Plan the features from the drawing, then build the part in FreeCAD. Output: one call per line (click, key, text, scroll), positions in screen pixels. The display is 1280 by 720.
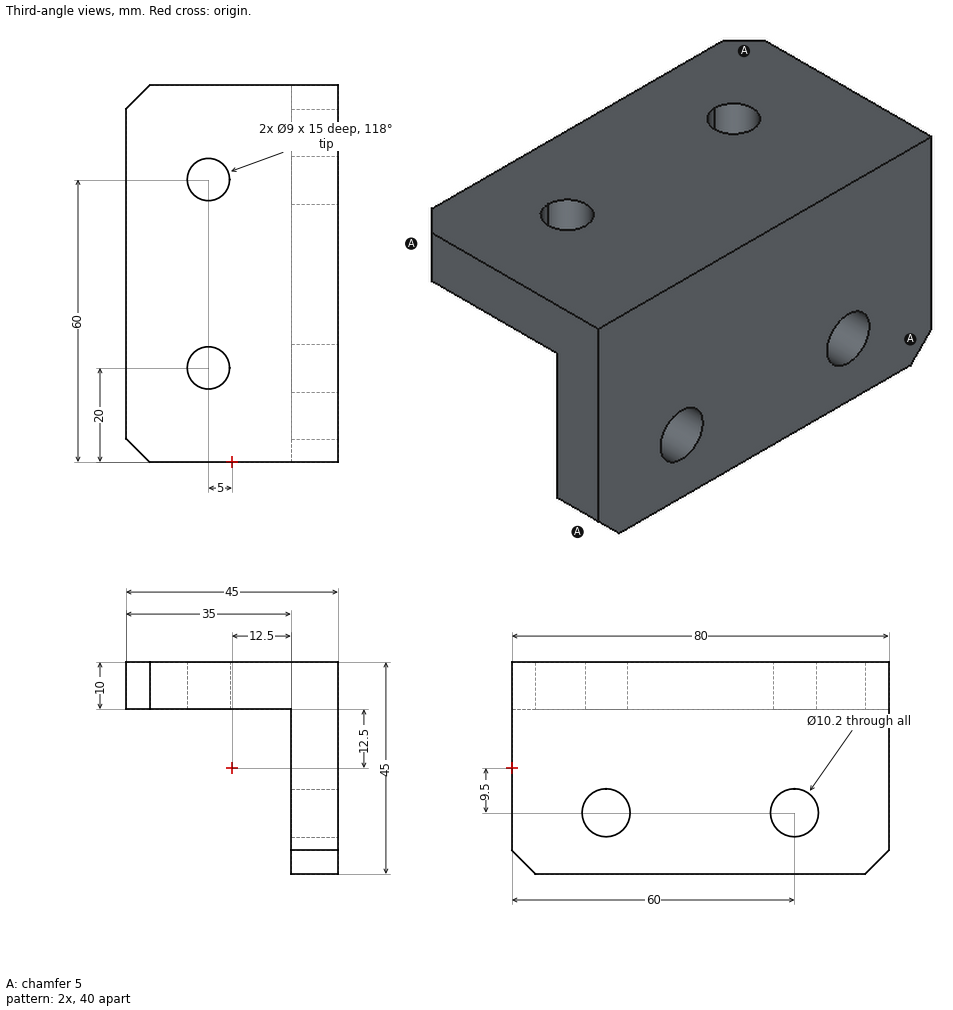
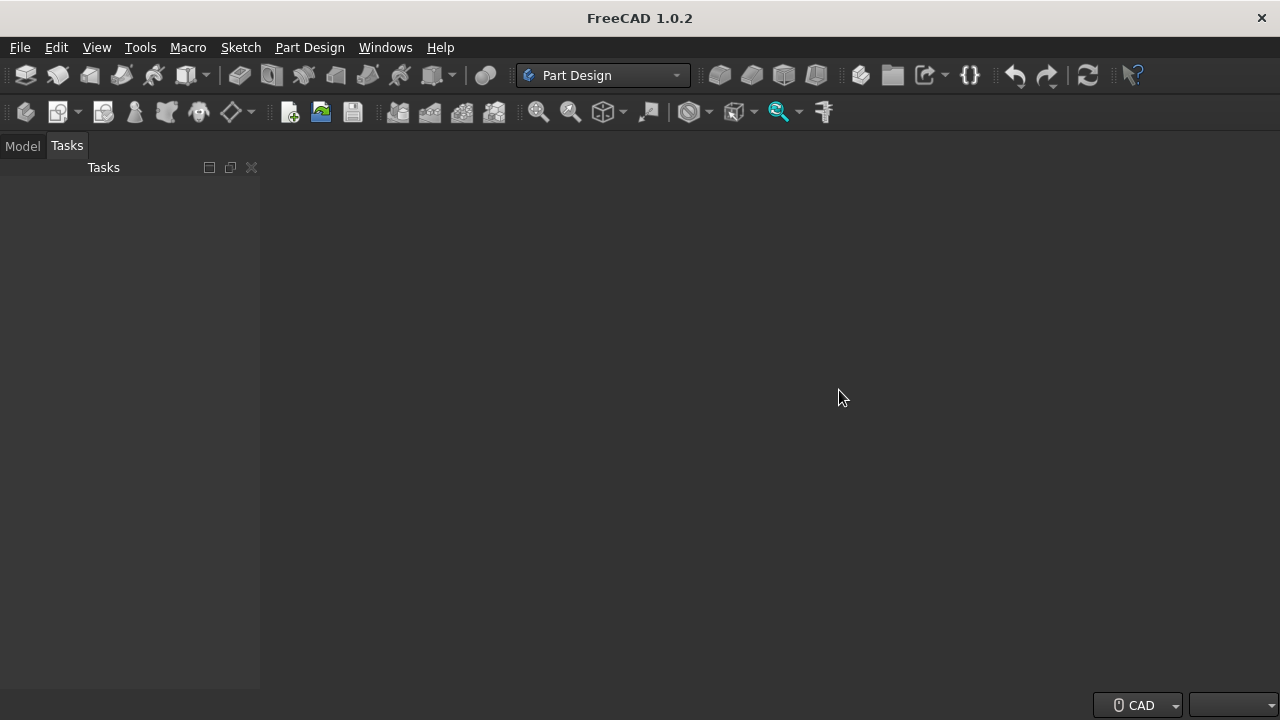
key(ctrl+n)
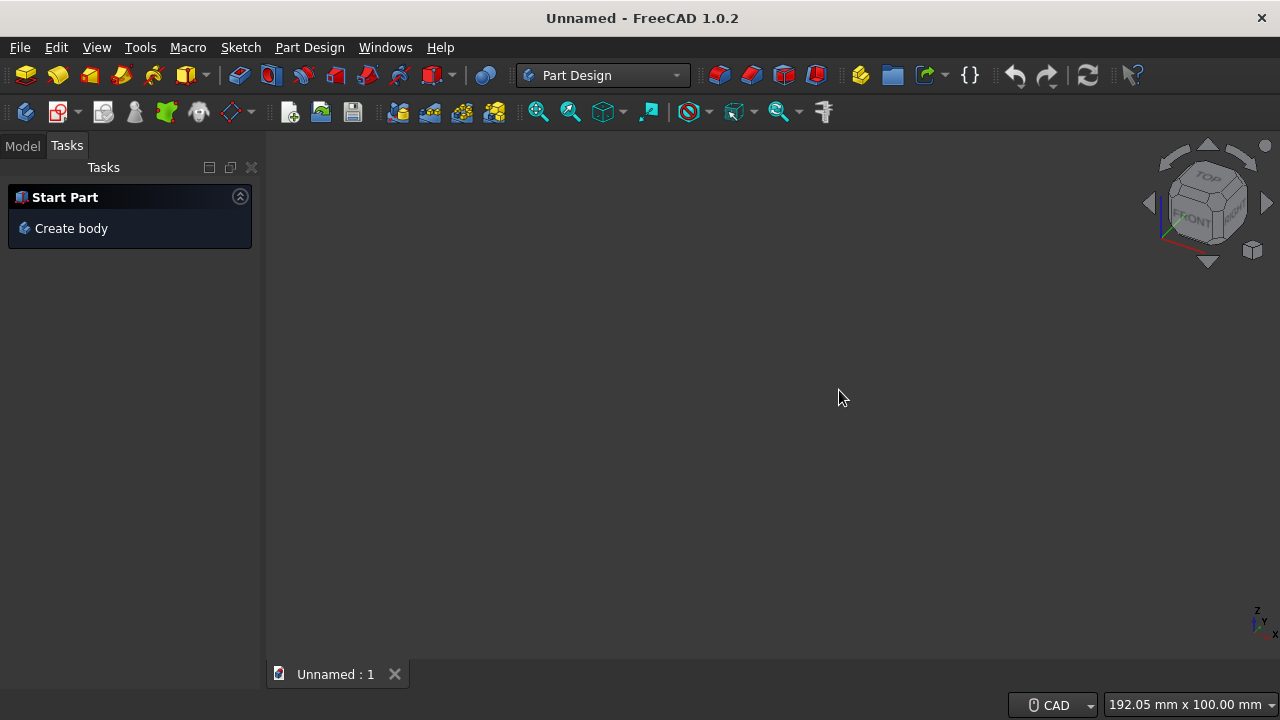
click(58, 112)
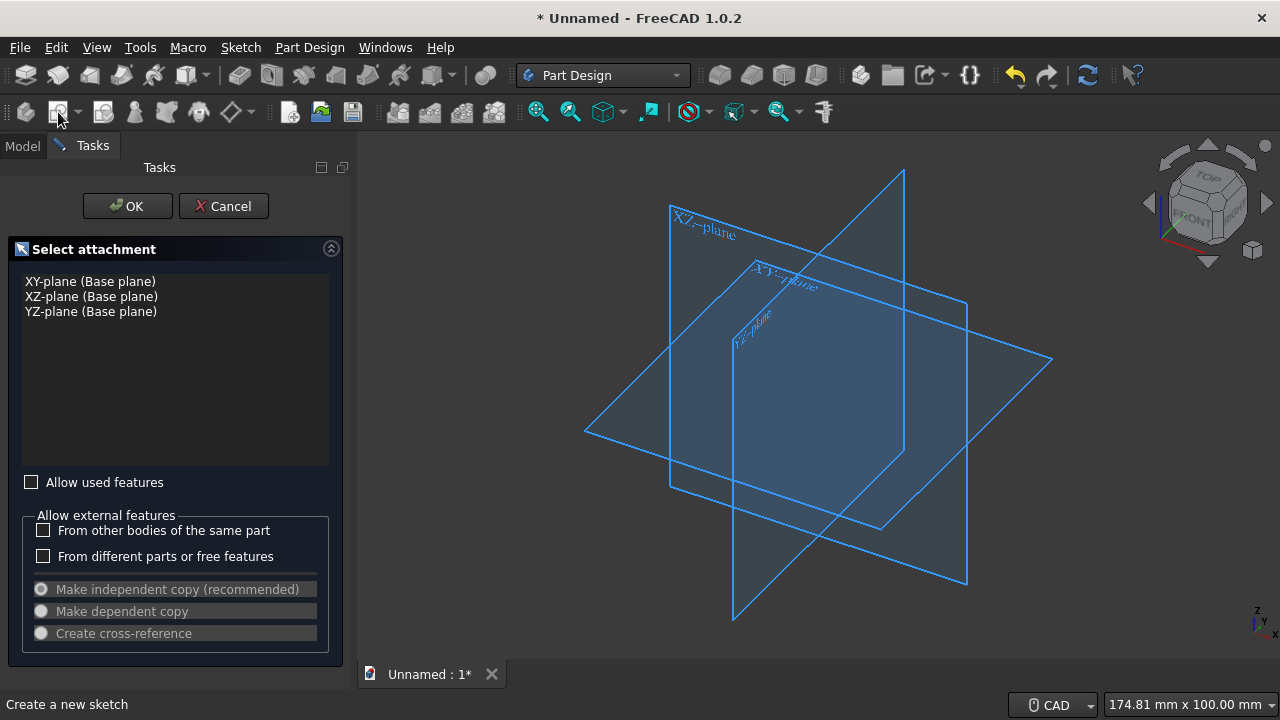
click(82, 296)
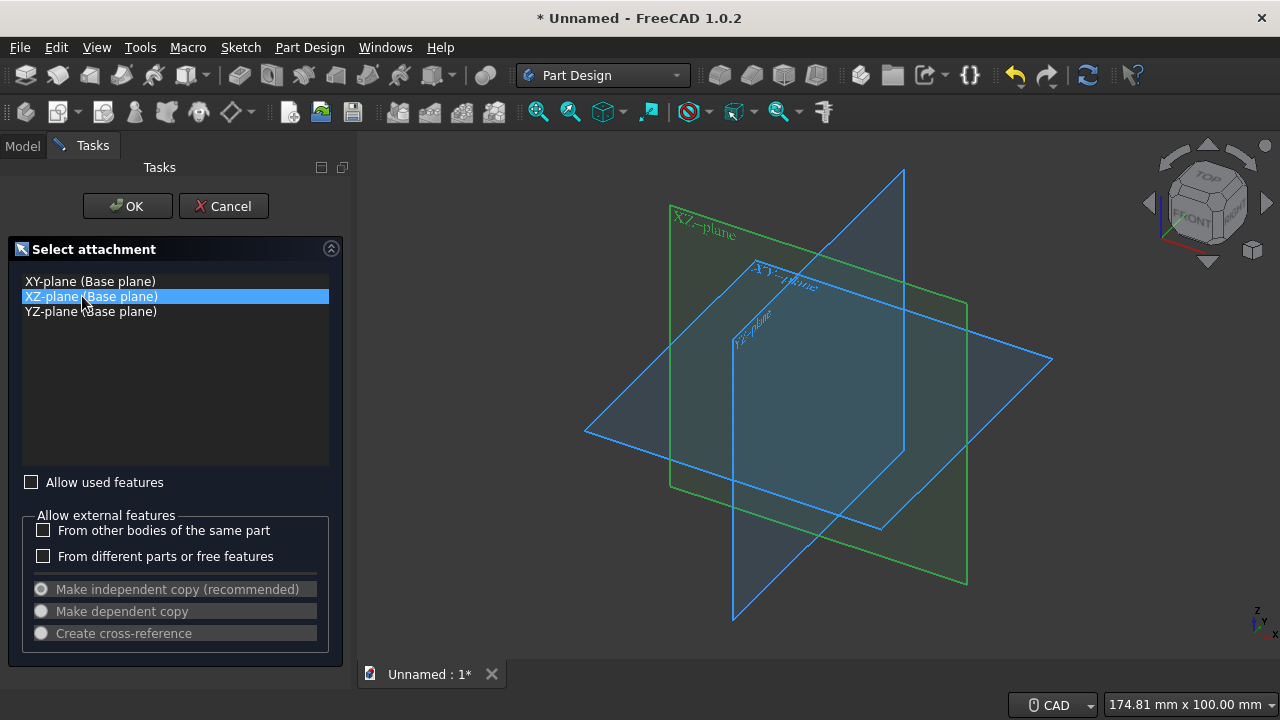
click(128, 206)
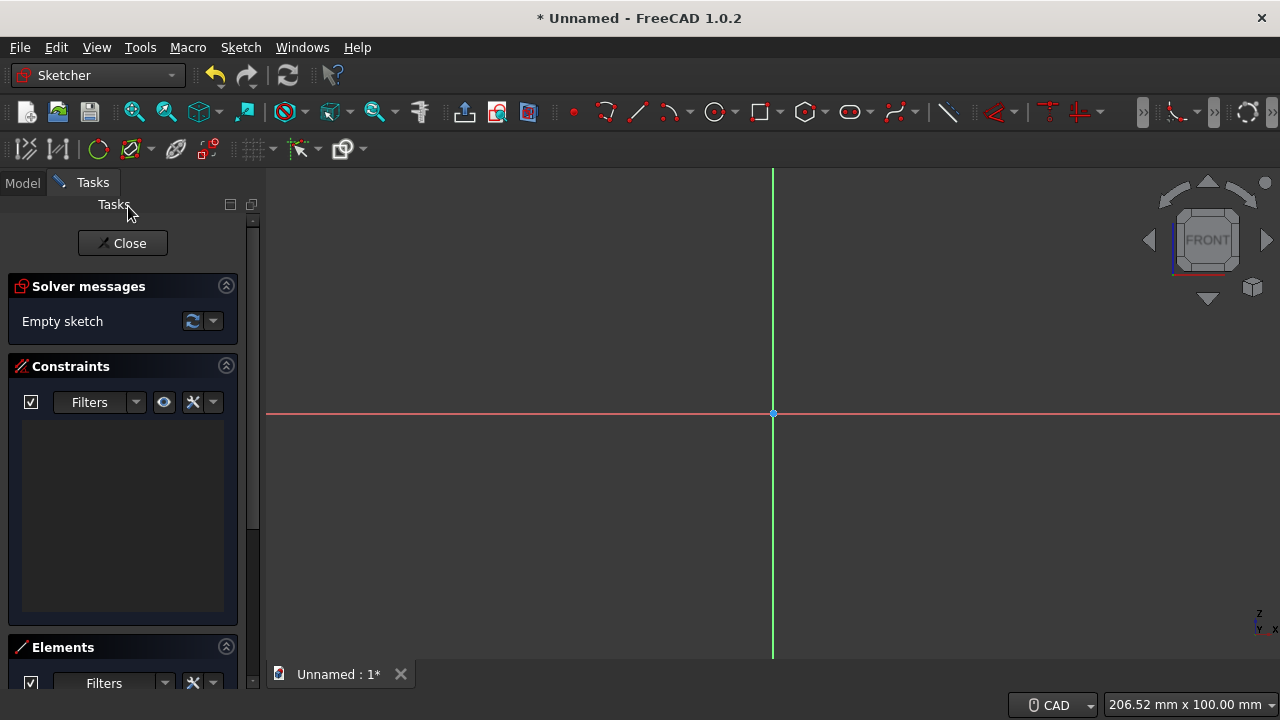
scroll(912, 413, up, 2)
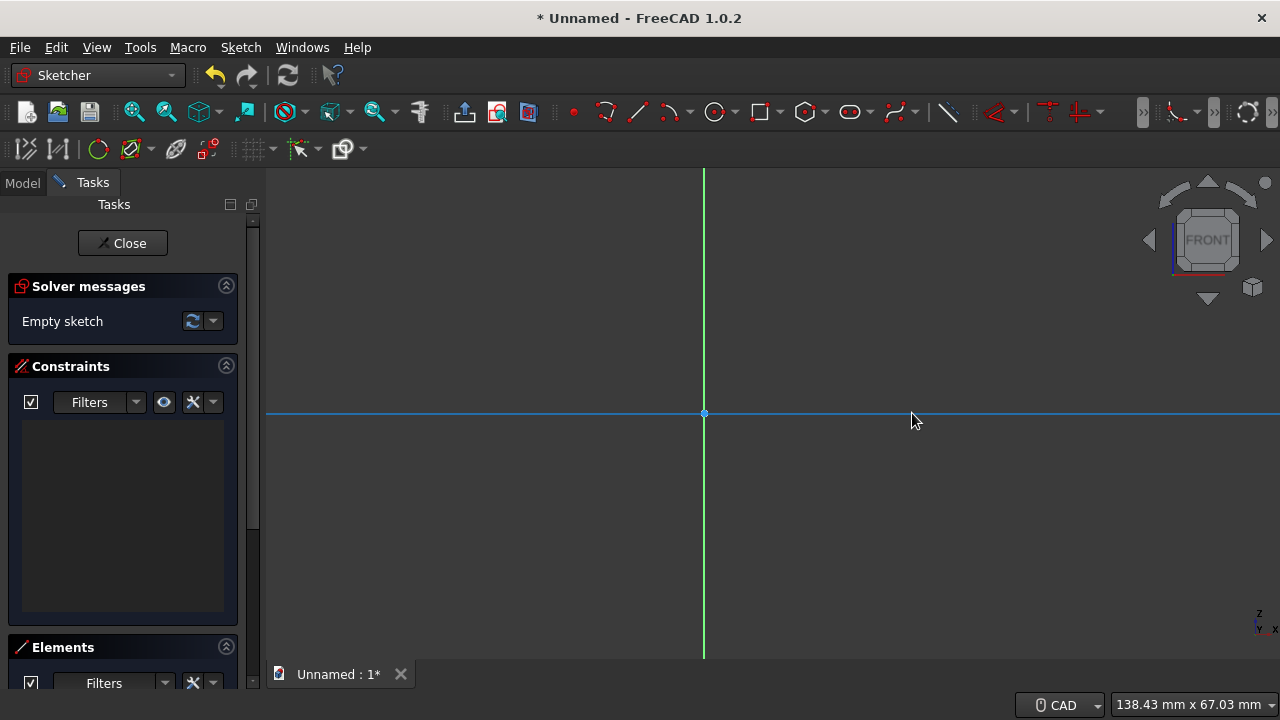
key(g)
key(m)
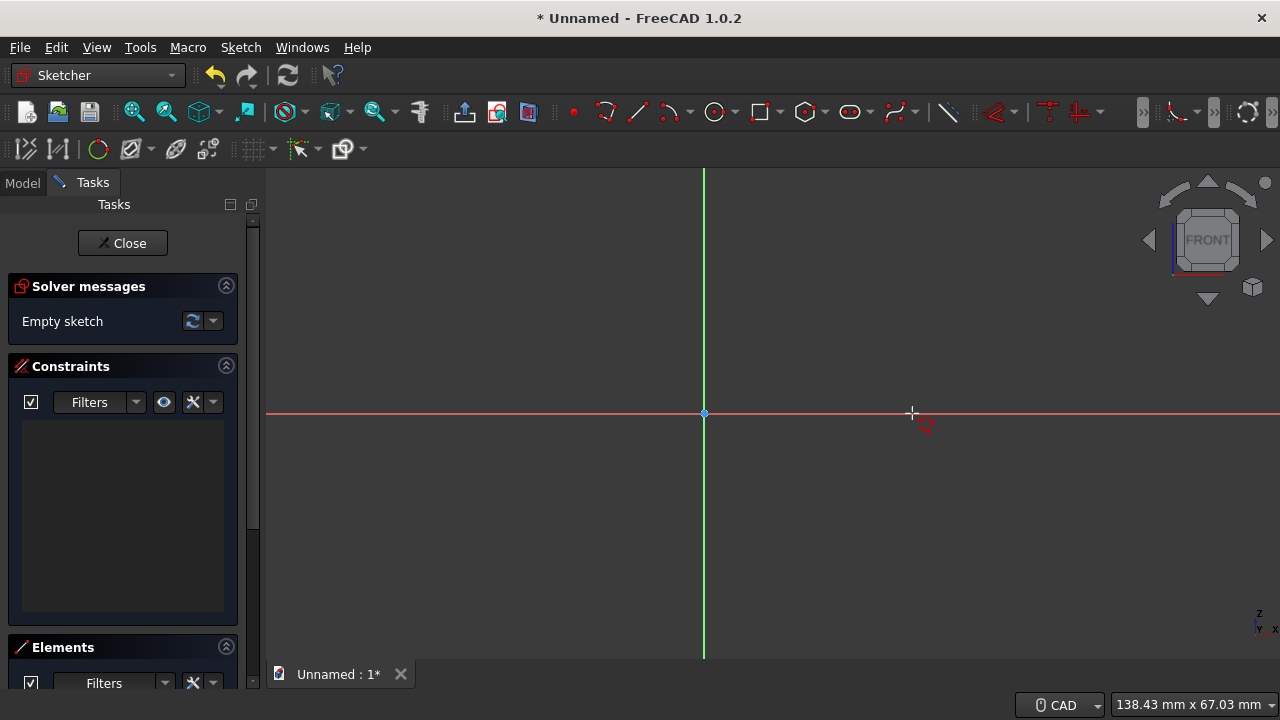
click(796, 322)
click(540, 322)
click(540, 249)
click(869, 249)
click(869, 578)
click(796, 578)
click(796, 323)
key(Escape)
key(Escape)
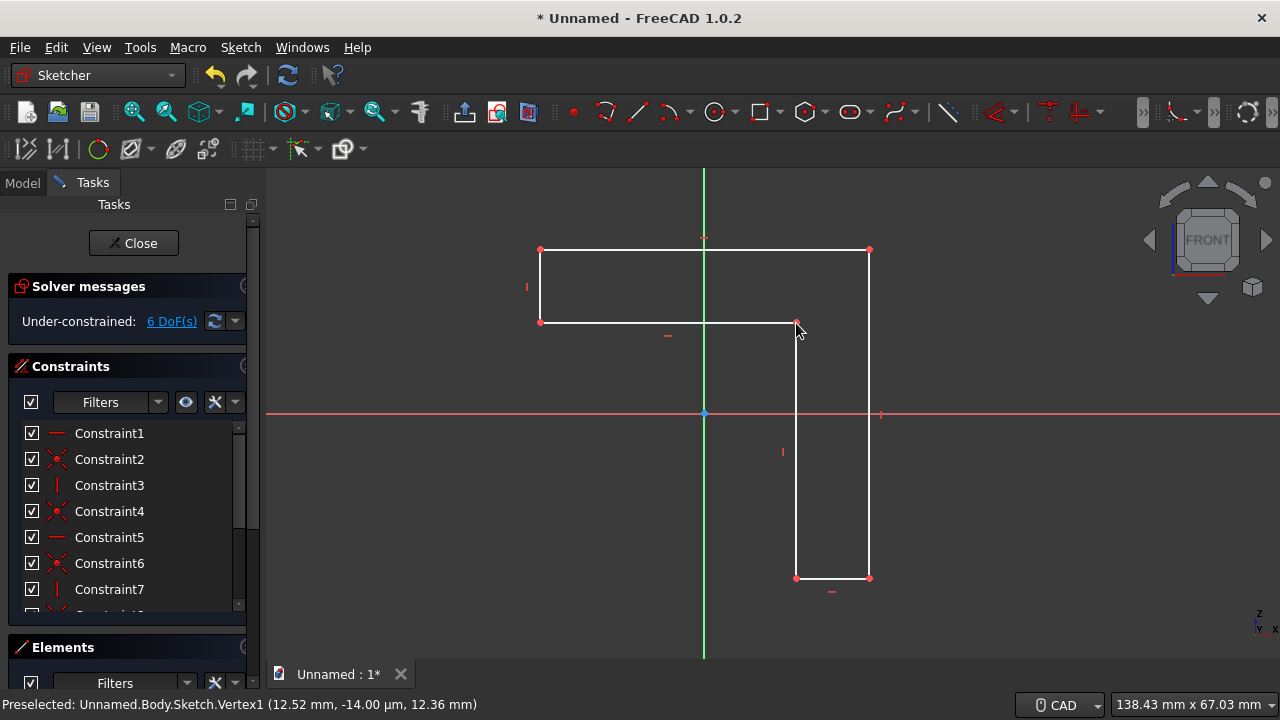
click(994, 112)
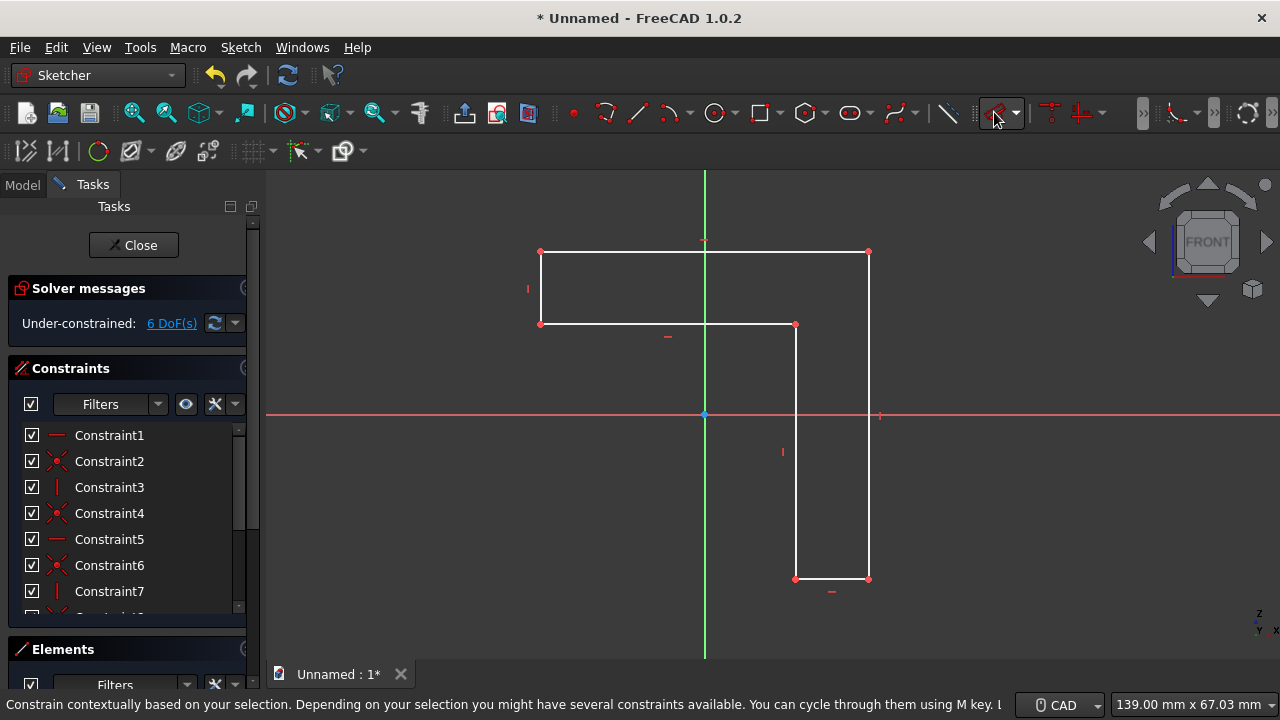
click(719, 324)
click(668, 290)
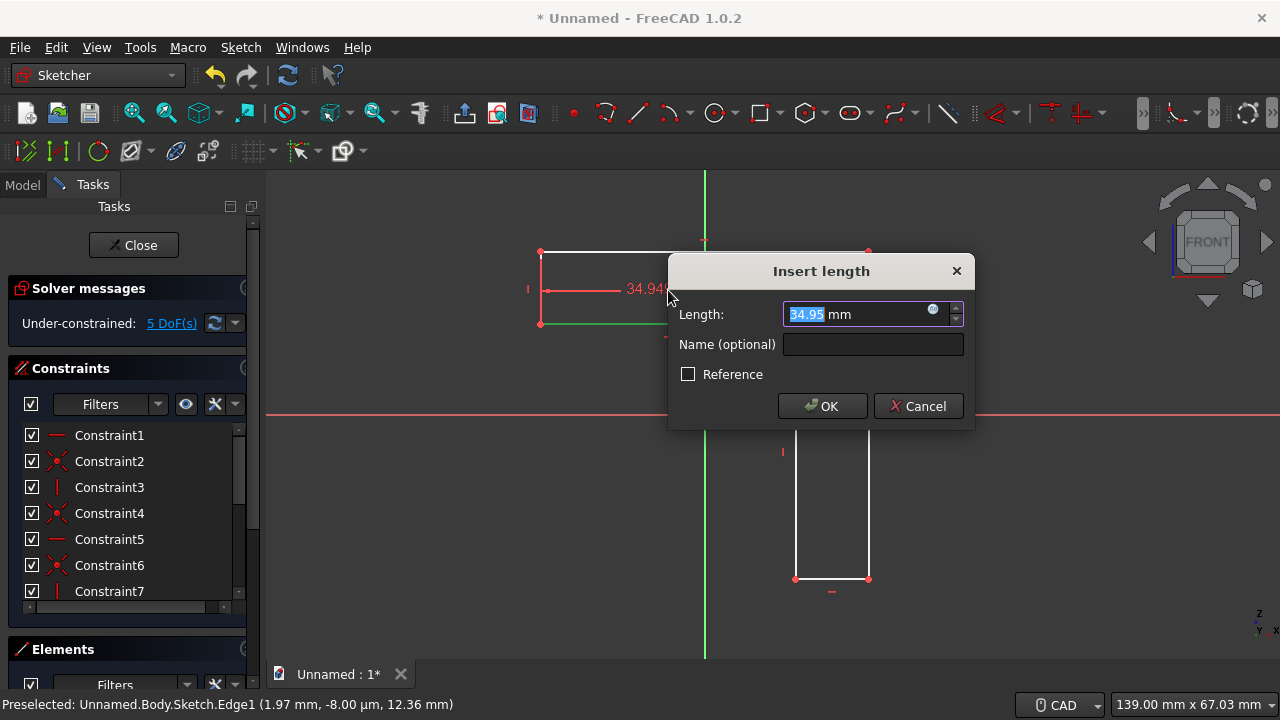
text(35)
key(Return)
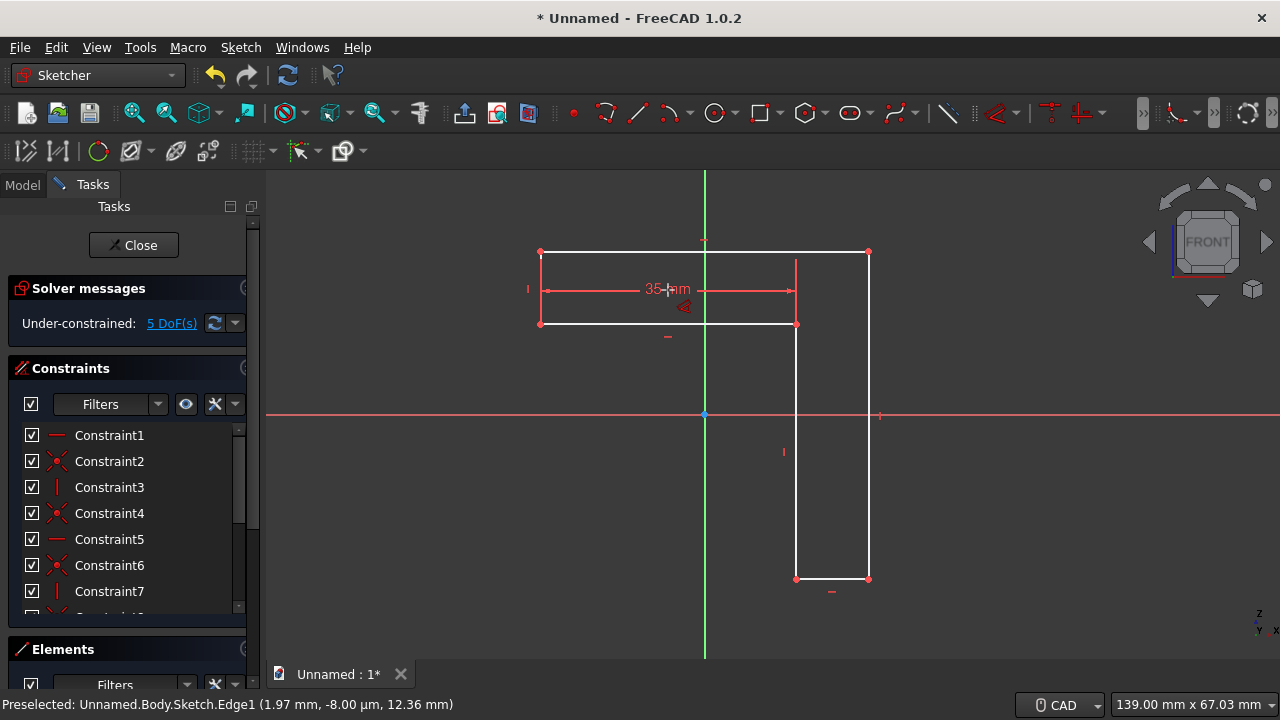
click(541, 303)
click(507, 288)